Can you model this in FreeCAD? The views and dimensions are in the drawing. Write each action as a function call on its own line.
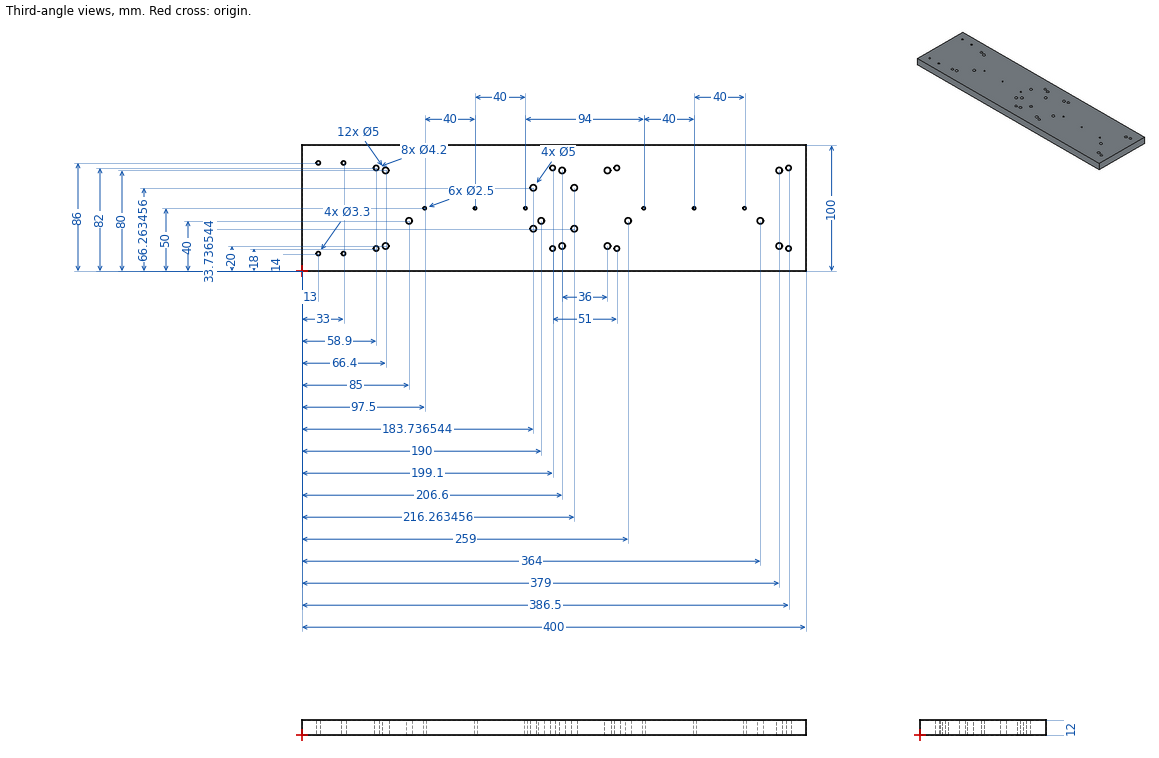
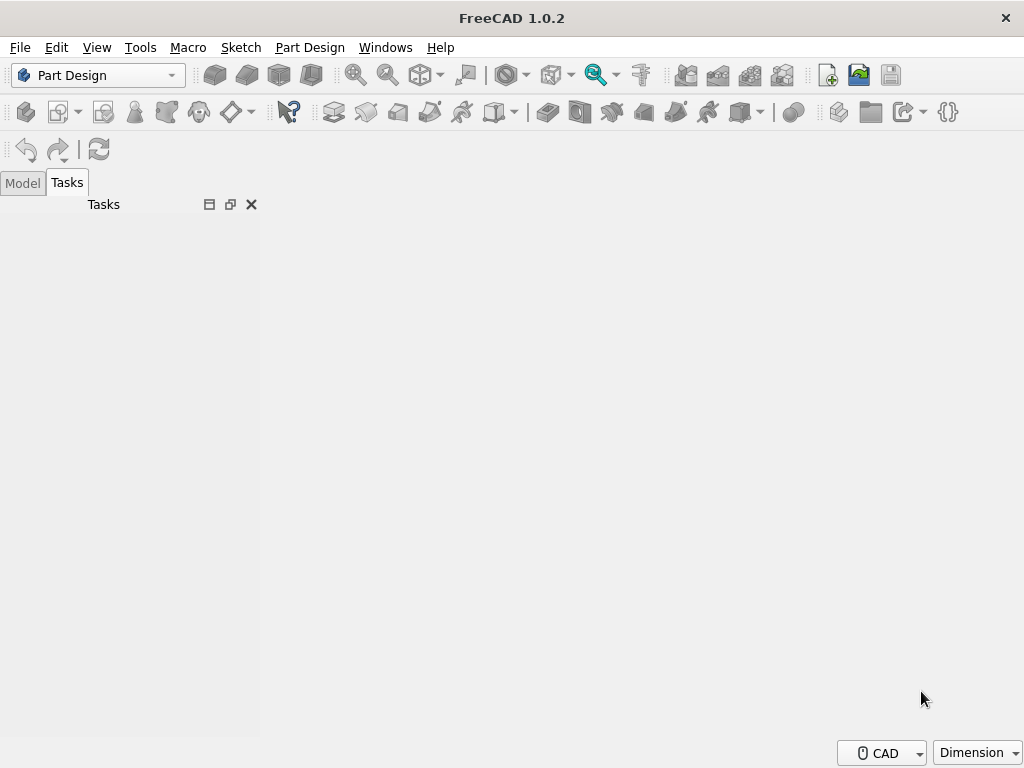
click(828, 76)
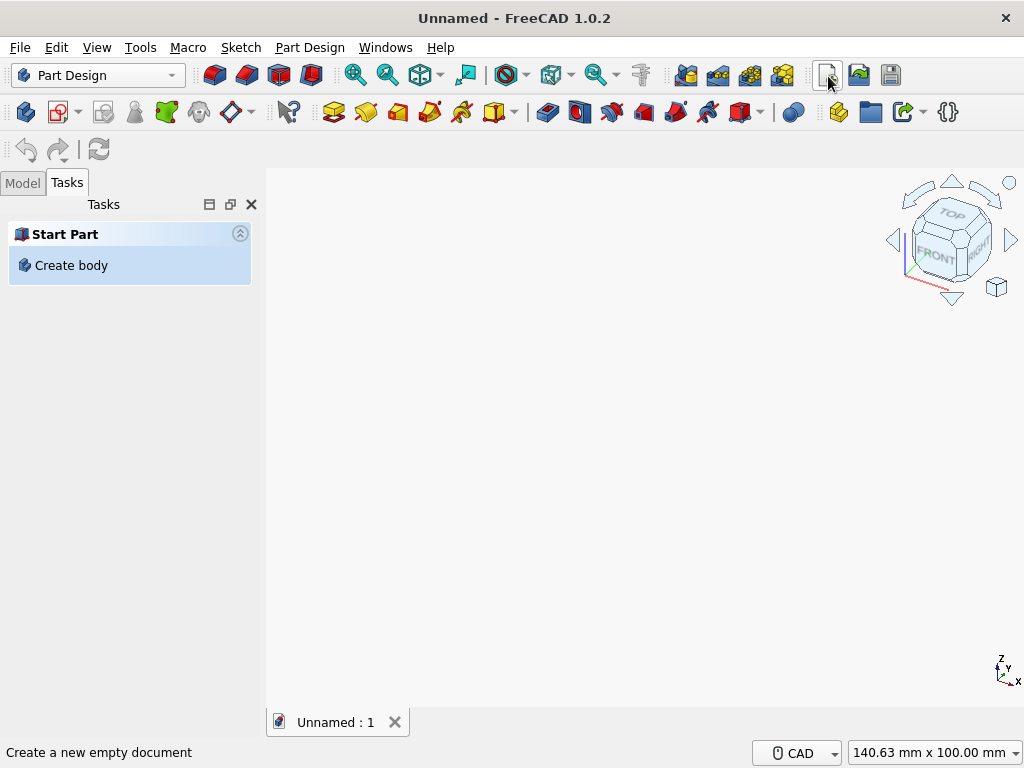
click(58, 112)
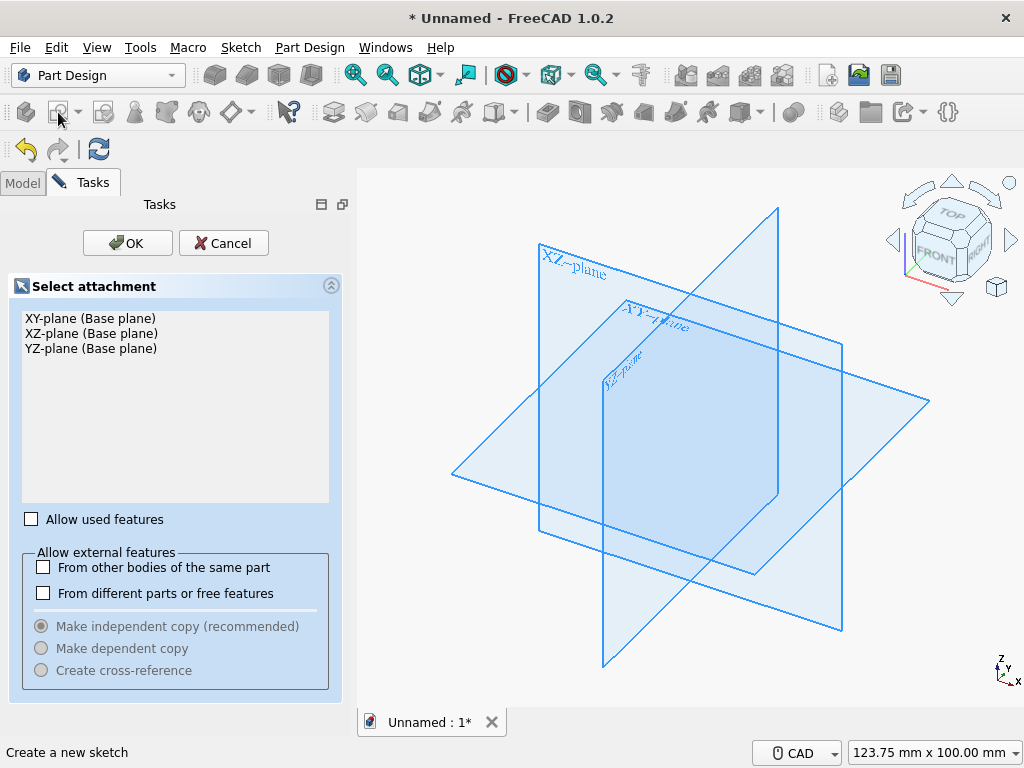
click(82, 318)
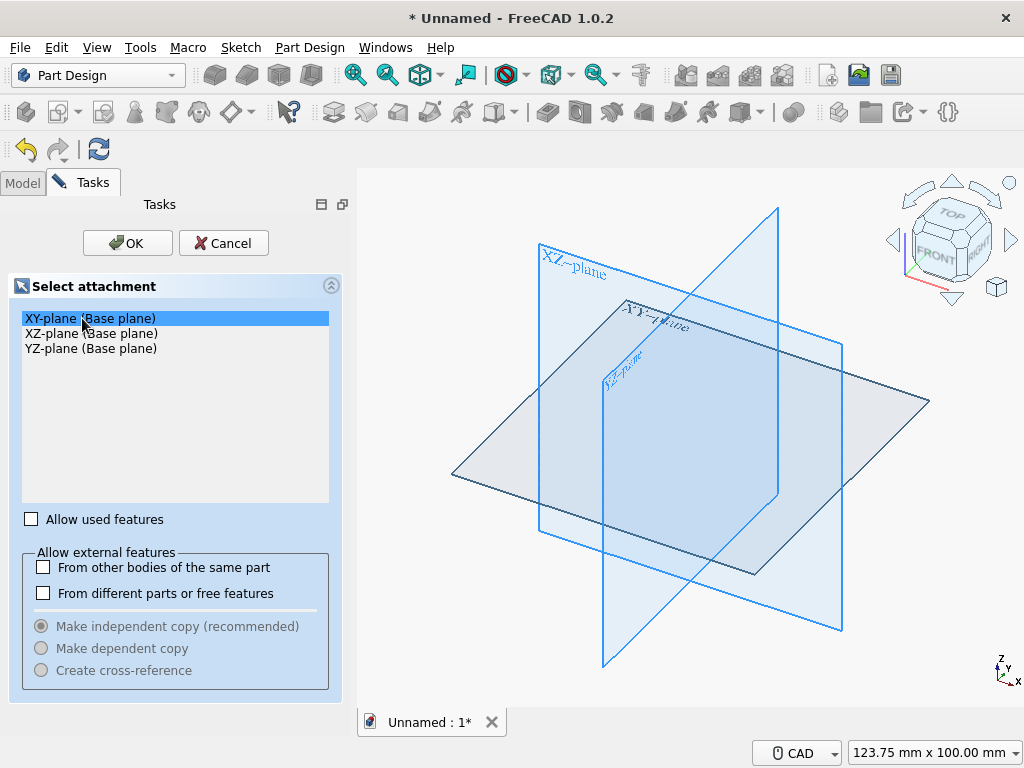
click(128, 243)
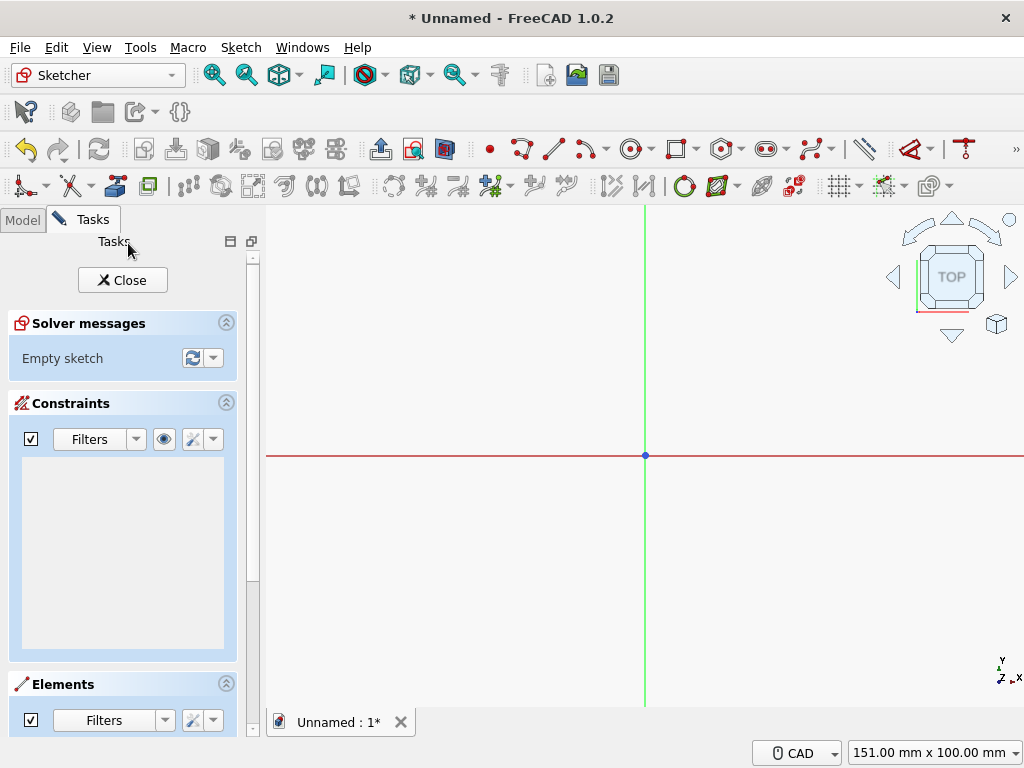
scroll(305, 519, down, 8)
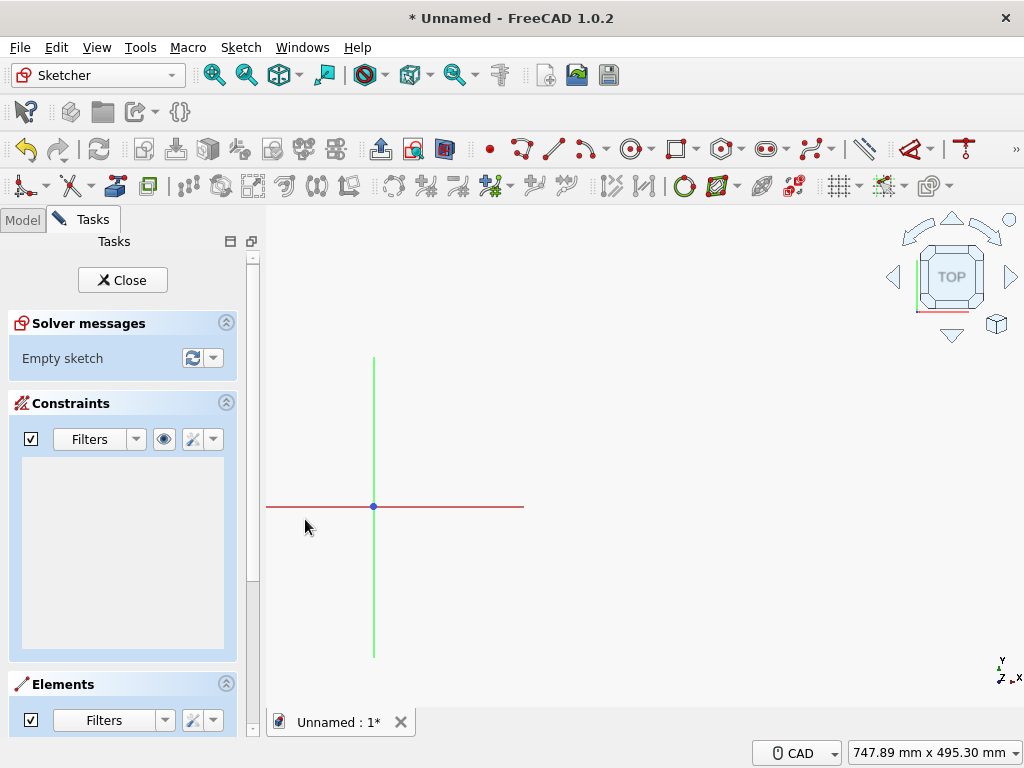
click(676, 150)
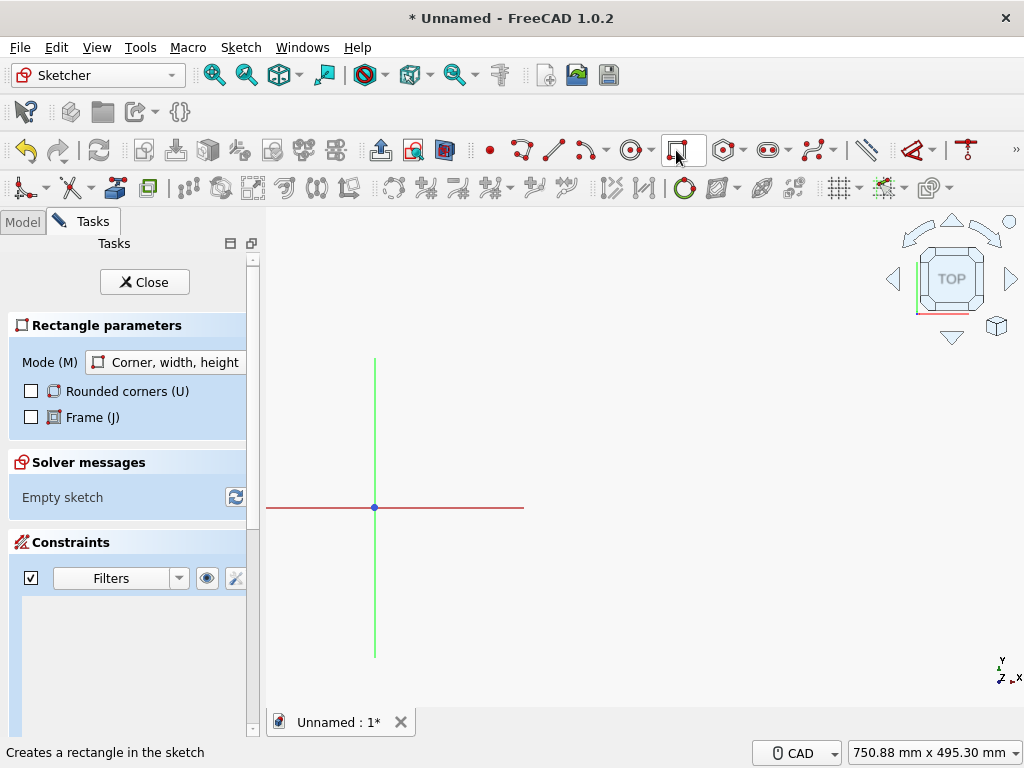
click(375, 508)
click(779, 407)
key(Escape)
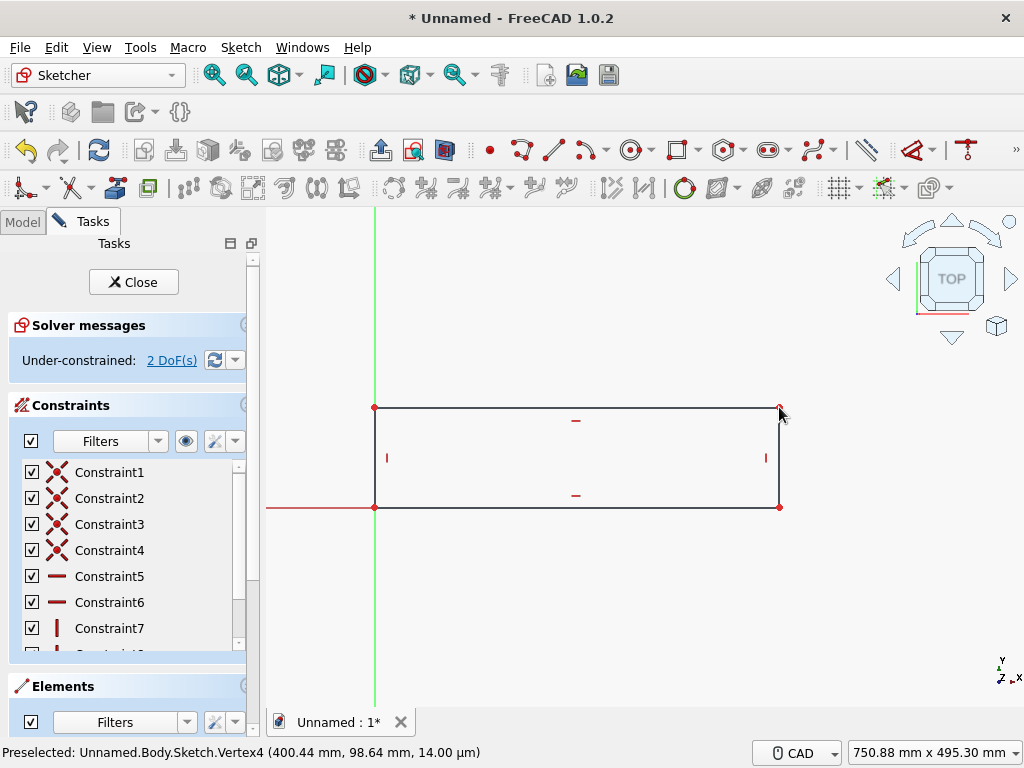
click(912, 150)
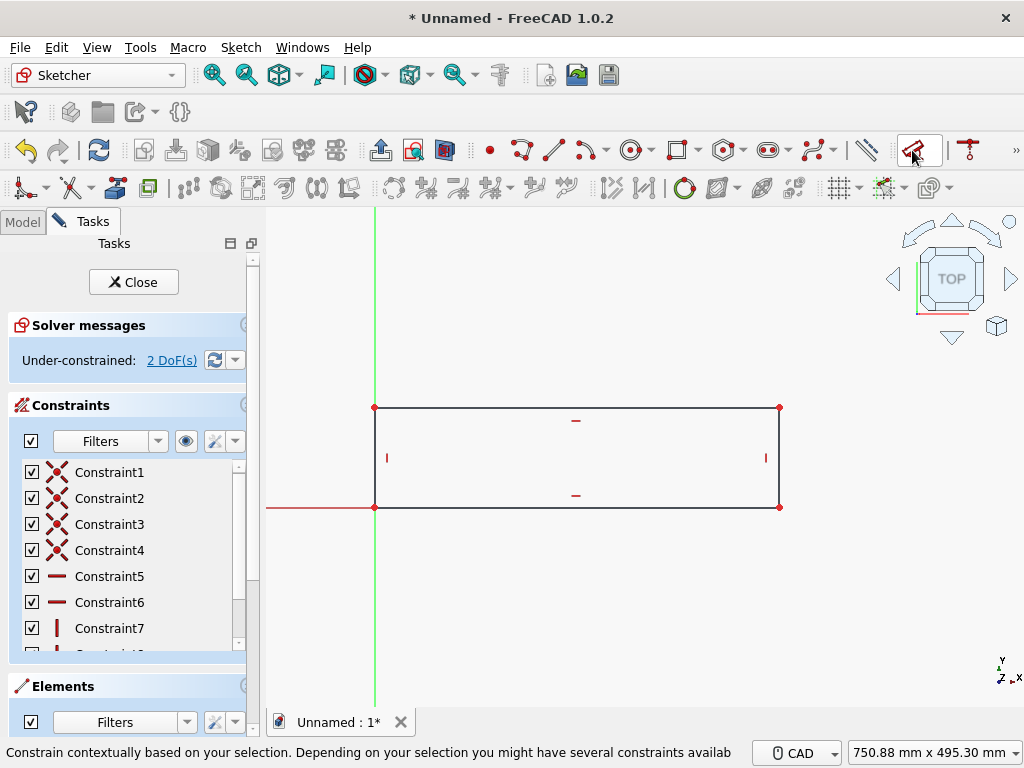
click(496, 508)
click(577, 542)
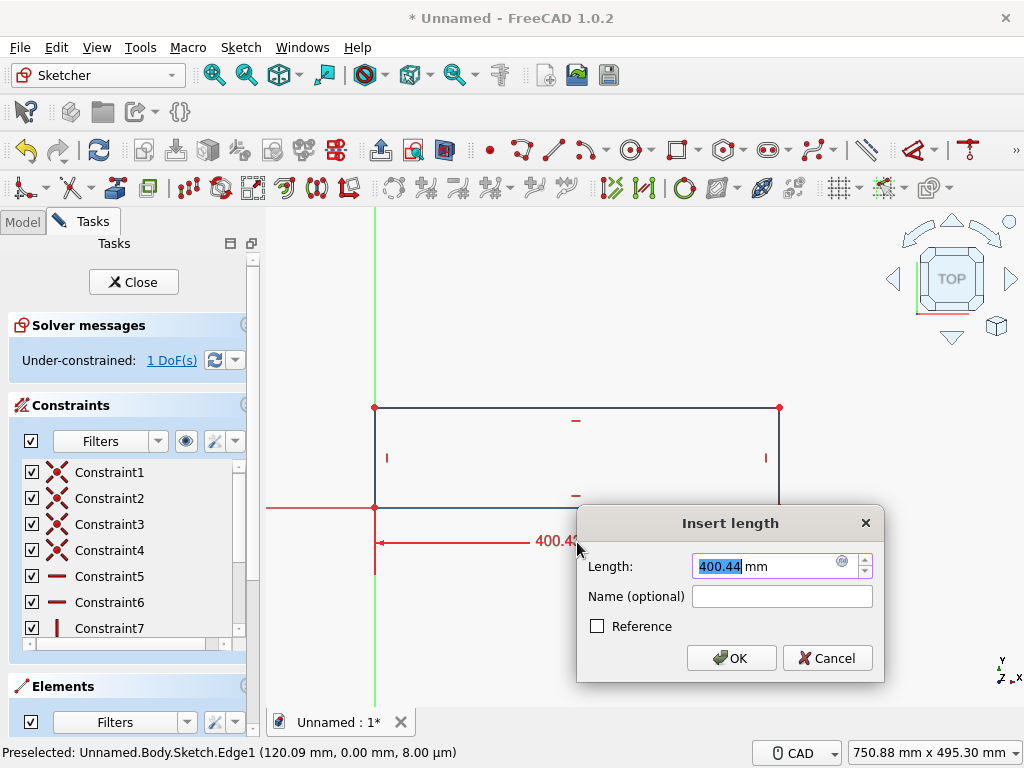
text(400)
key(Return)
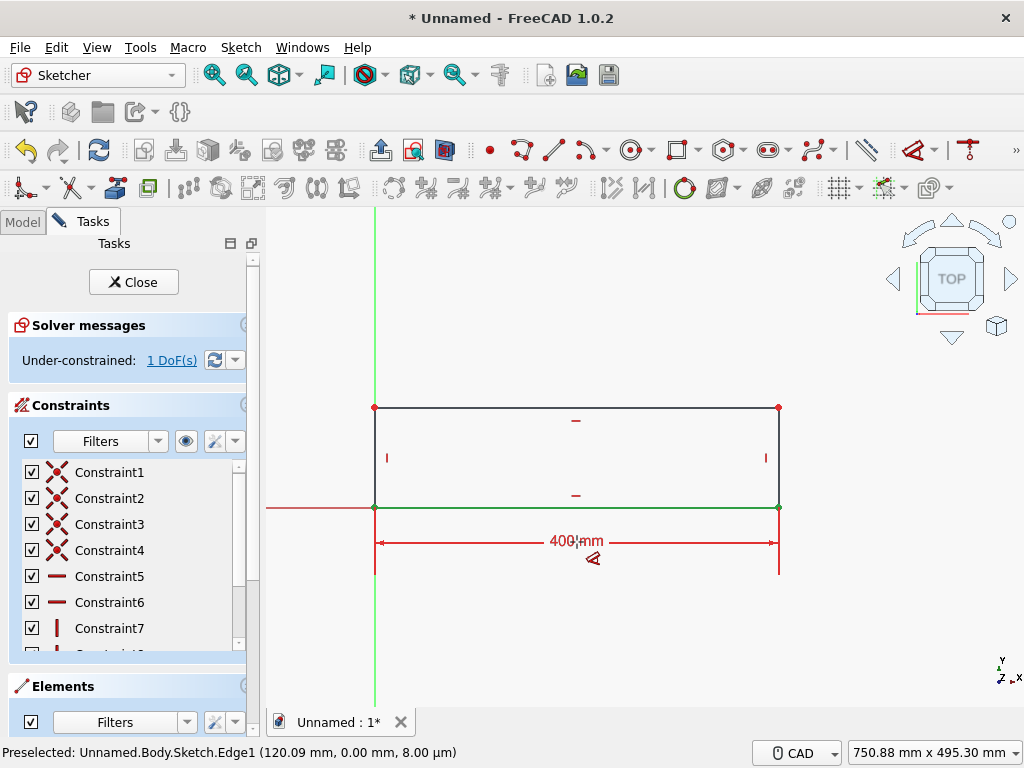
click(779, 478)
click(813, 458)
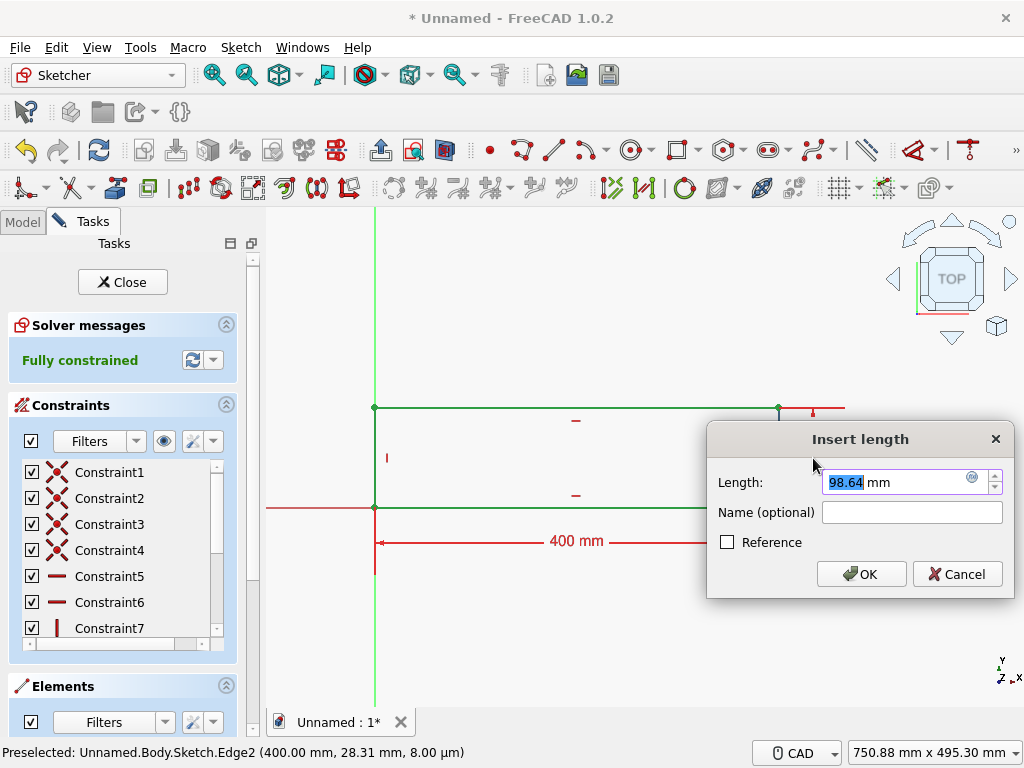
text(100)
key(Return)
key(Escape)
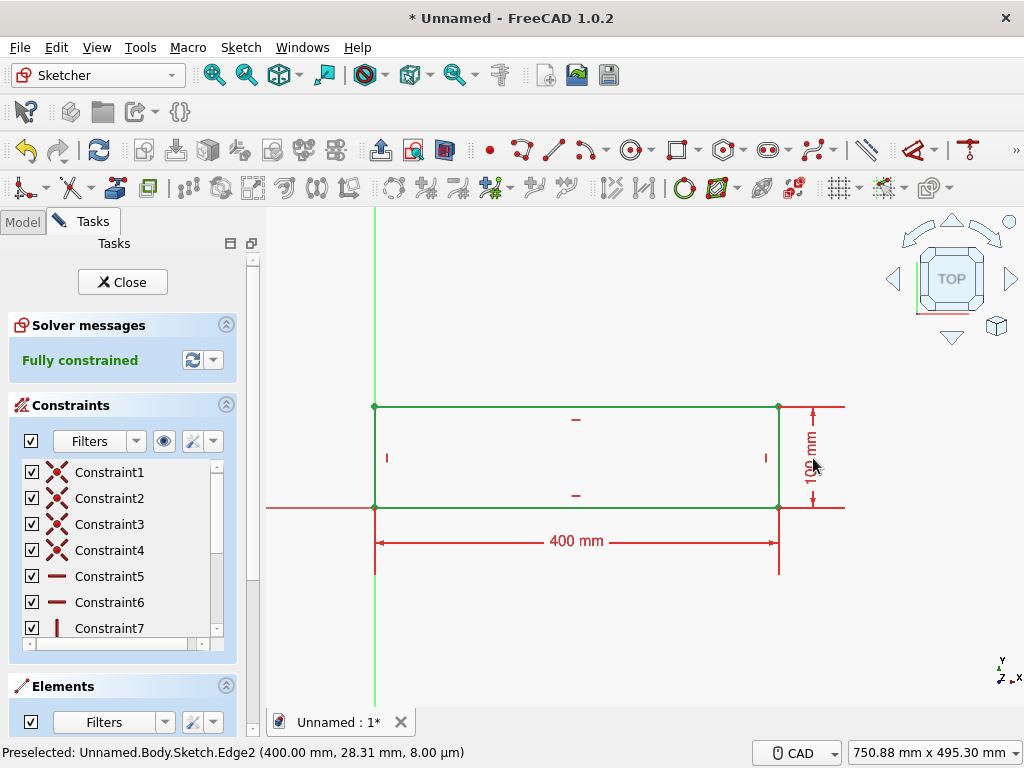
click(123, 282)